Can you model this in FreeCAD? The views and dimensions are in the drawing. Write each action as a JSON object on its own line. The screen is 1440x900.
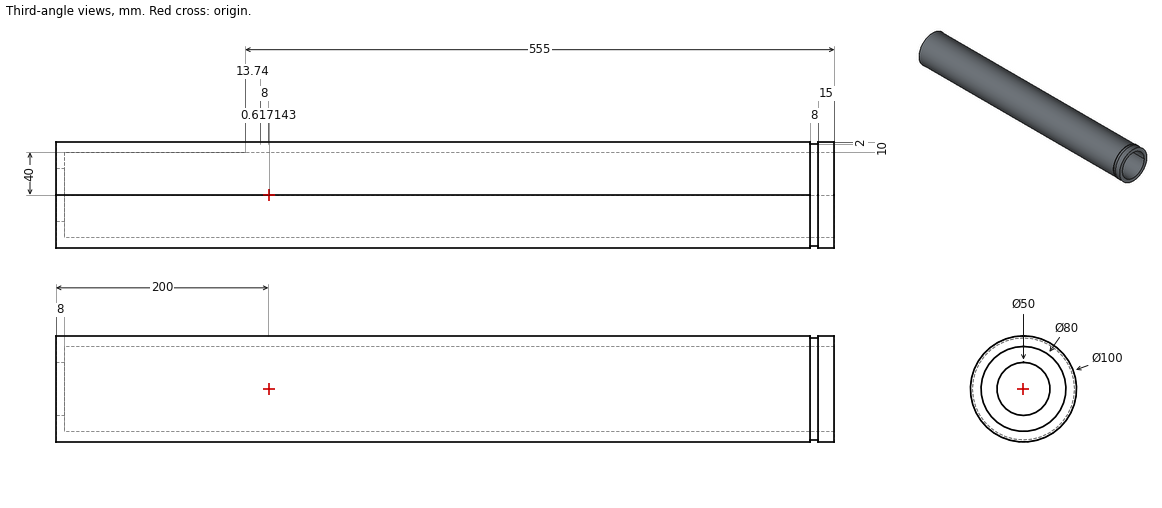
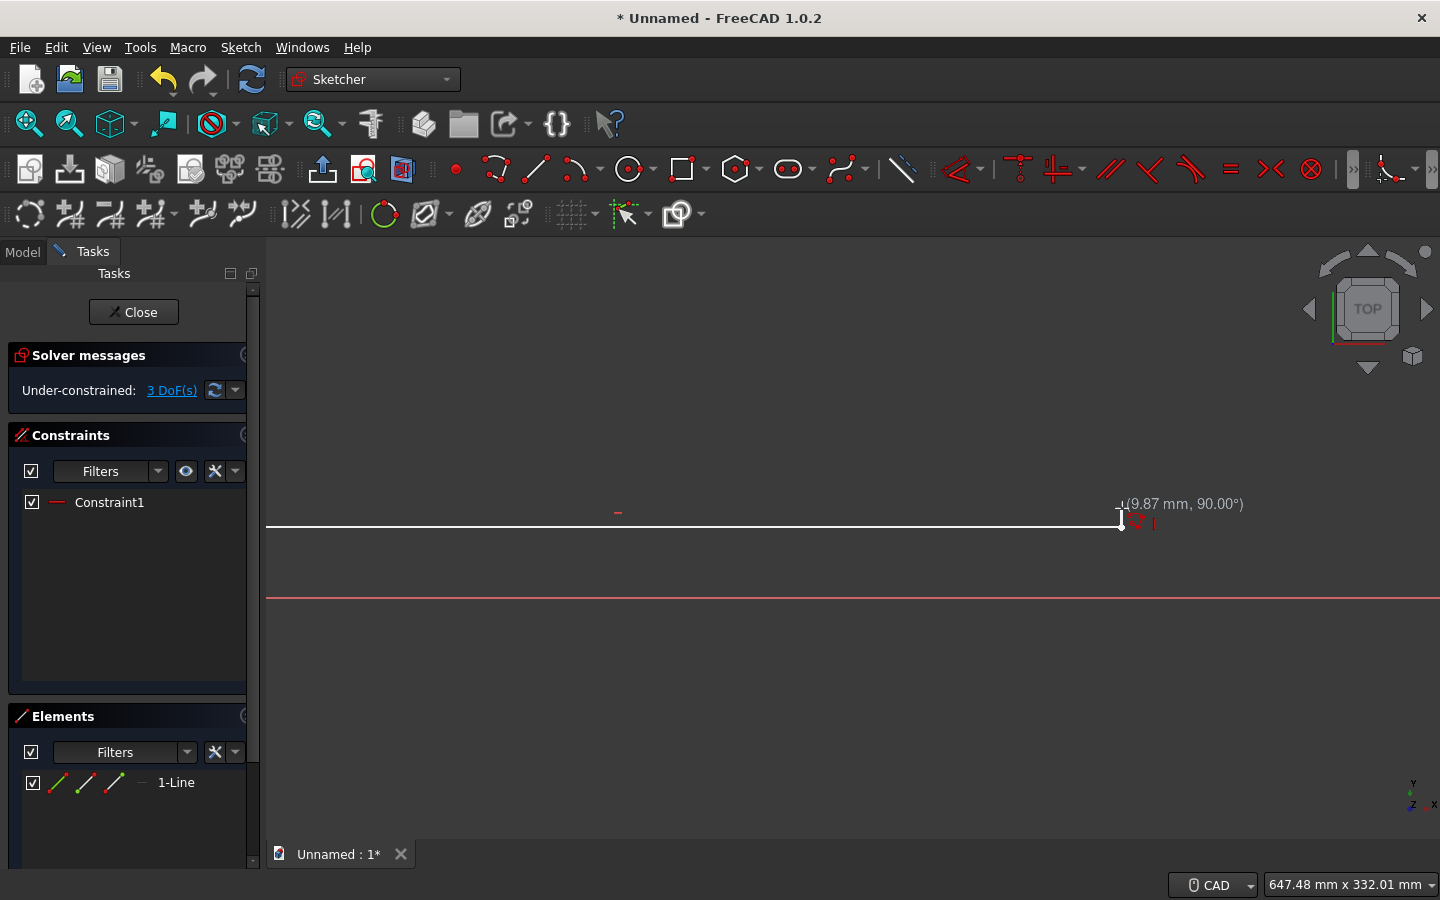
{"action": "left_click", "coordinate": [1122, 508]}
{"action": "left_click", "coordinate": [1095, 508]}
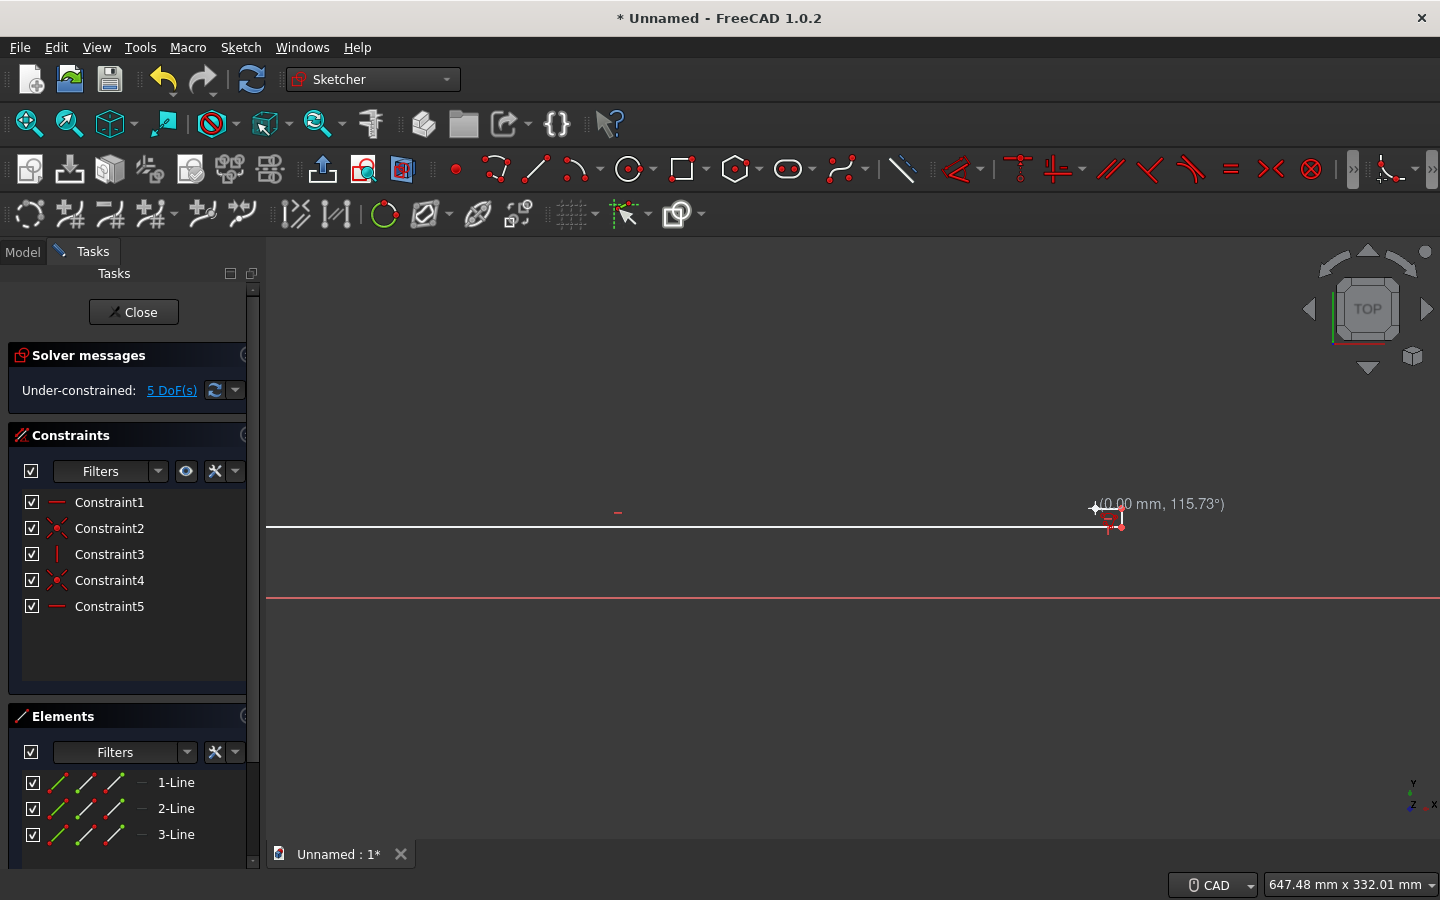
{"action": "scroll", "coordinate": [1095, 511], "scroll_direction": "up", "scroll_amount": 8}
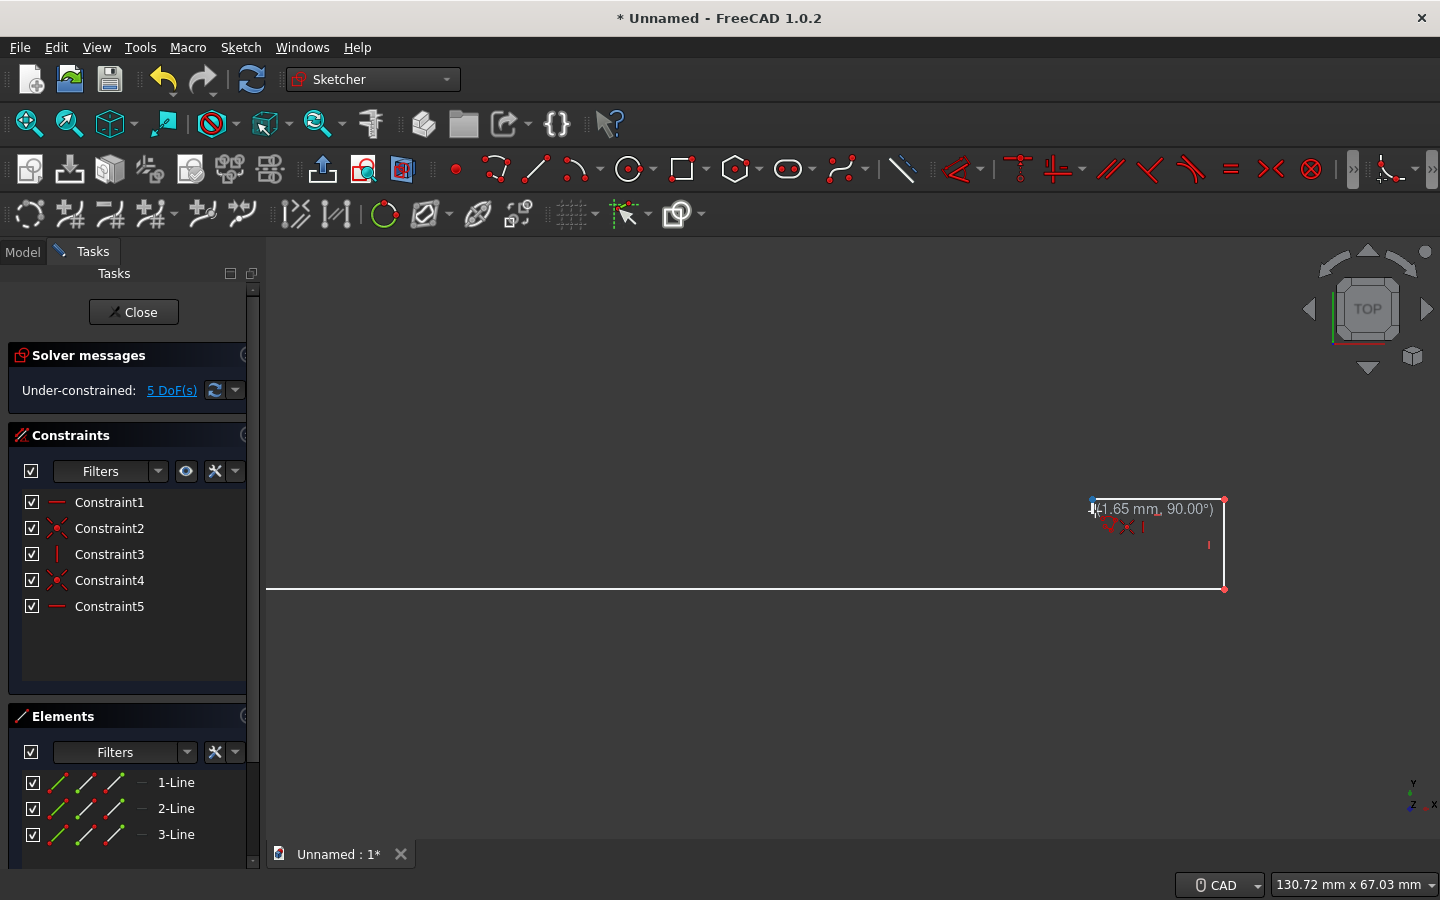
{"action": "left_click", "coordinate": [1092, 511]}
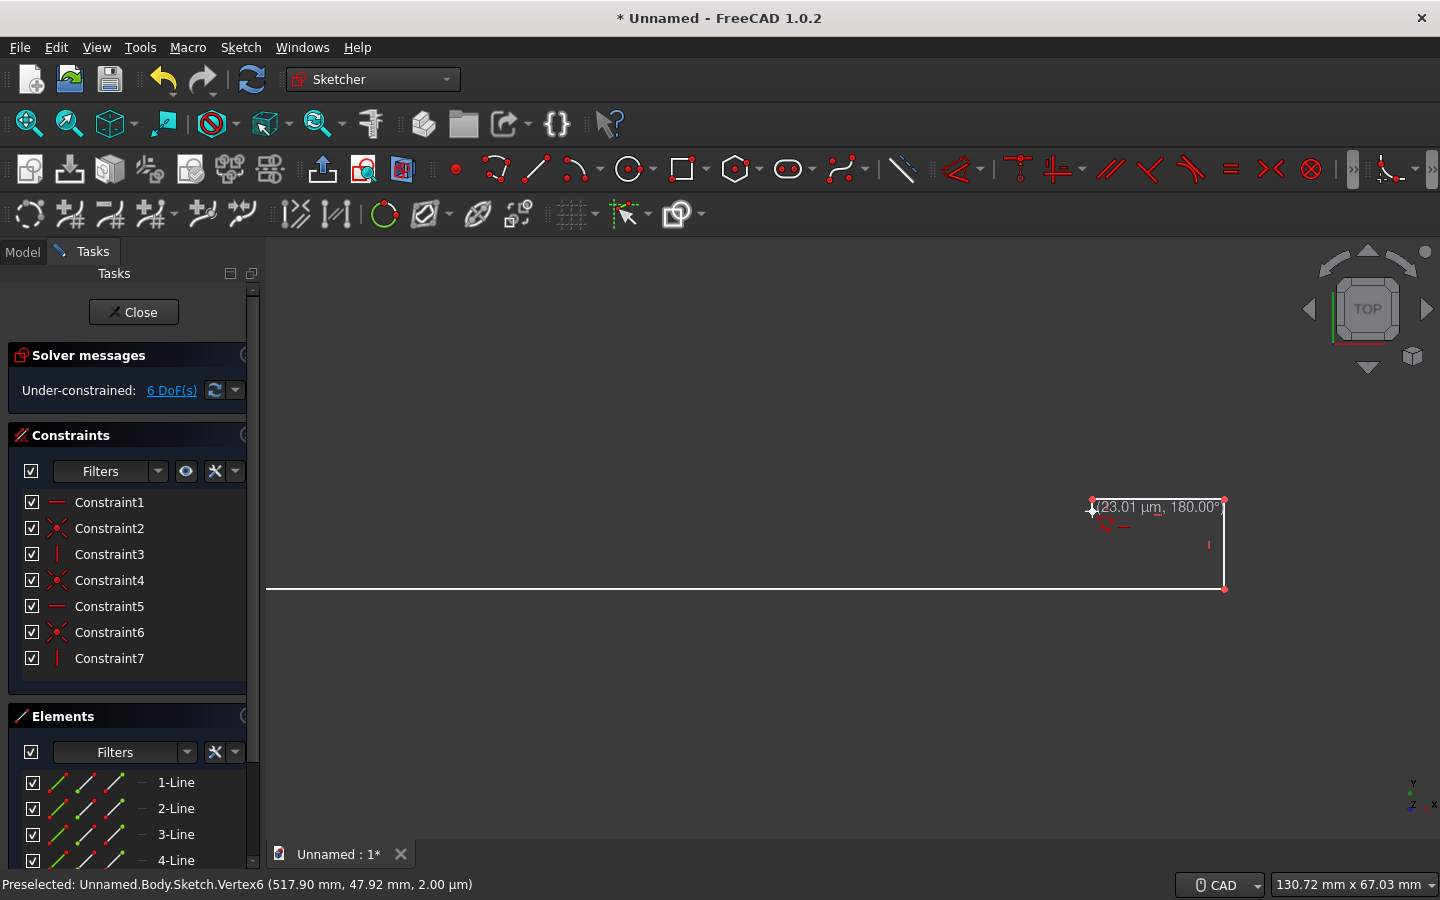
{"action": "scroll", "coordinate": [1106, 510], "scroll_direction": "down", "scroll_amount": 10}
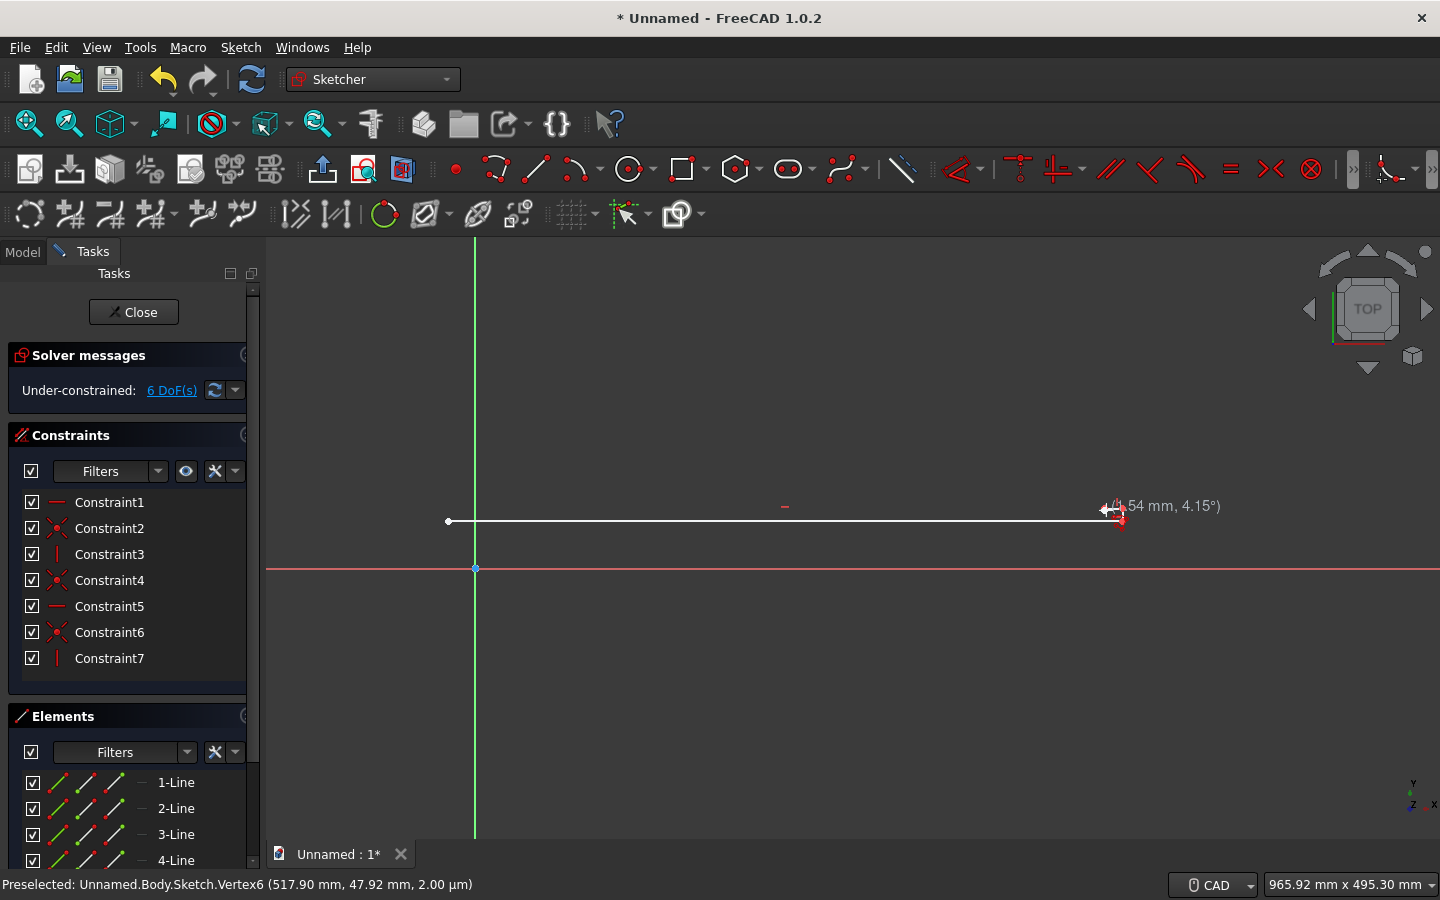
{"action": "scroll", "coordinate": [1095, 511], "scroll_direction": "up", "scroll_amount": 3}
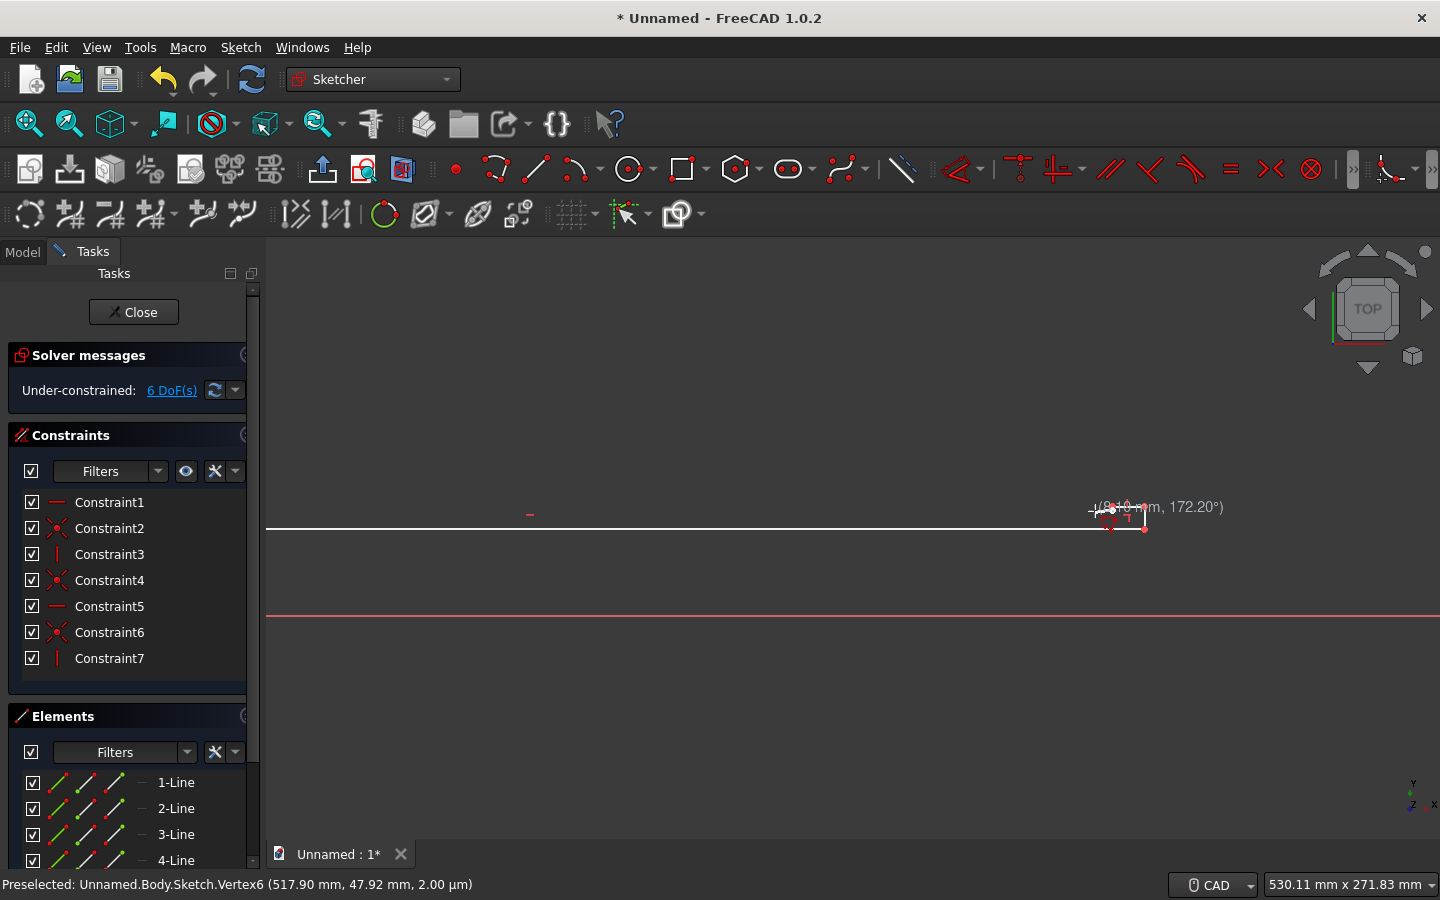
{"action": "left_click", "coordinate": [1094, 510]}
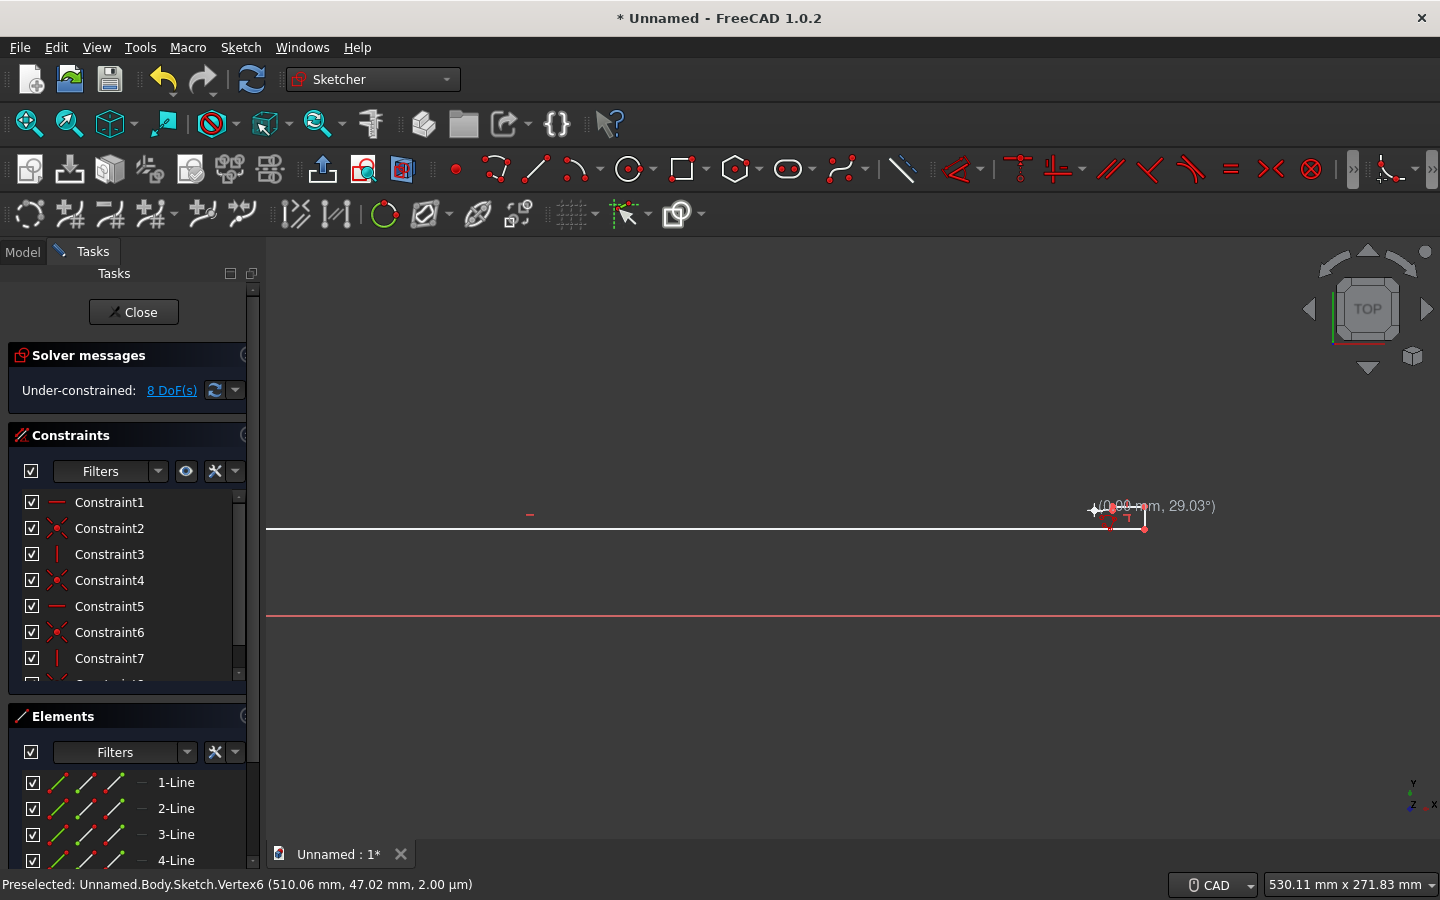
{"action": "scroll", "coordinate": [1094, 505], "scroll_direction": "up", "scroll_amount": 7}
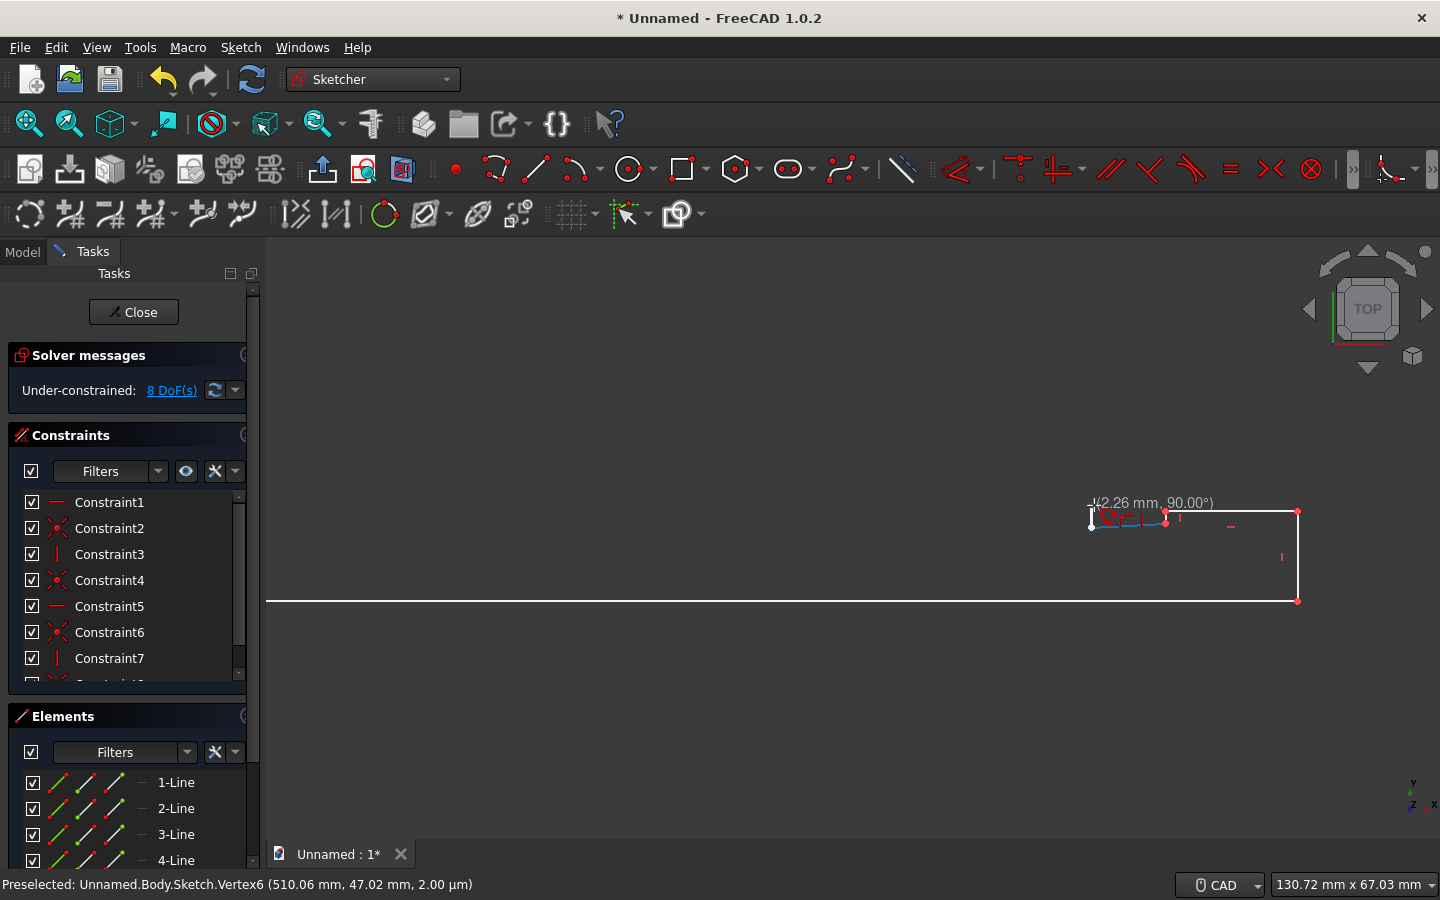
{"action": "left_click", "coordinate": [1092, 505]}